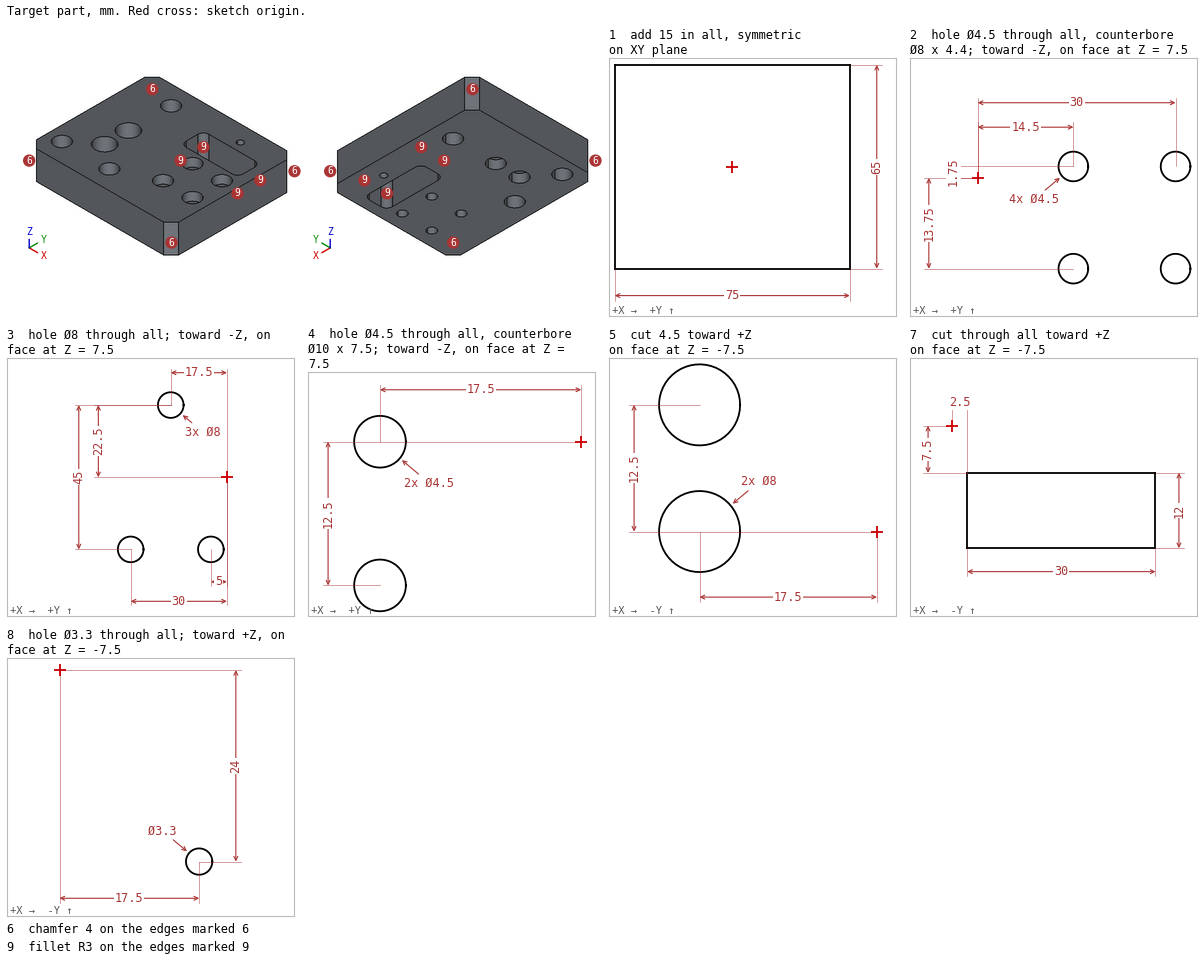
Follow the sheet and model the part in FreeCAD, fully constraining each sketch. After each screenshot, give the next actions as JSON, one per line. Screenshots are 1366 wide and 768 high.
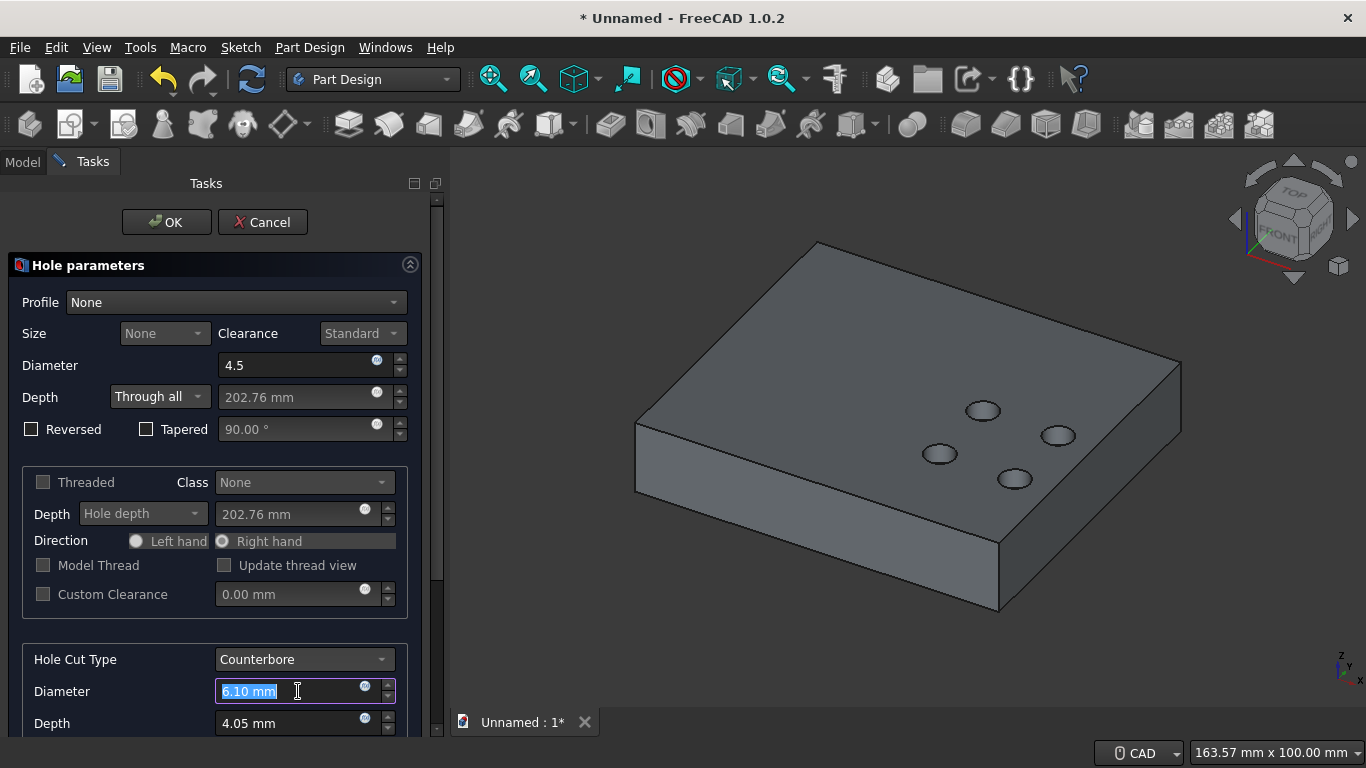
{"action": "type", "text": "8"}
{"action": "key", "text": "Tab"}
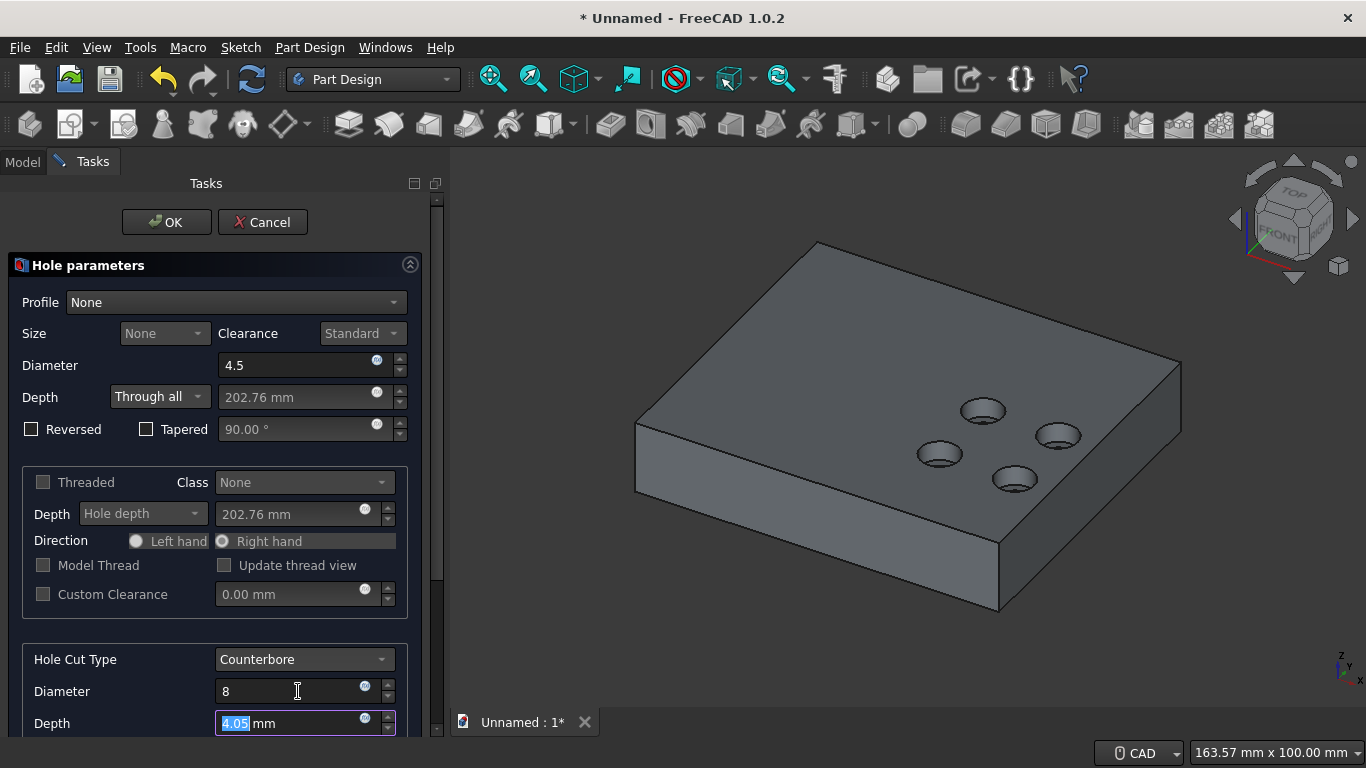
{"action": "type", "text": "4.4"}
{"action": "key", "text": "Tab"}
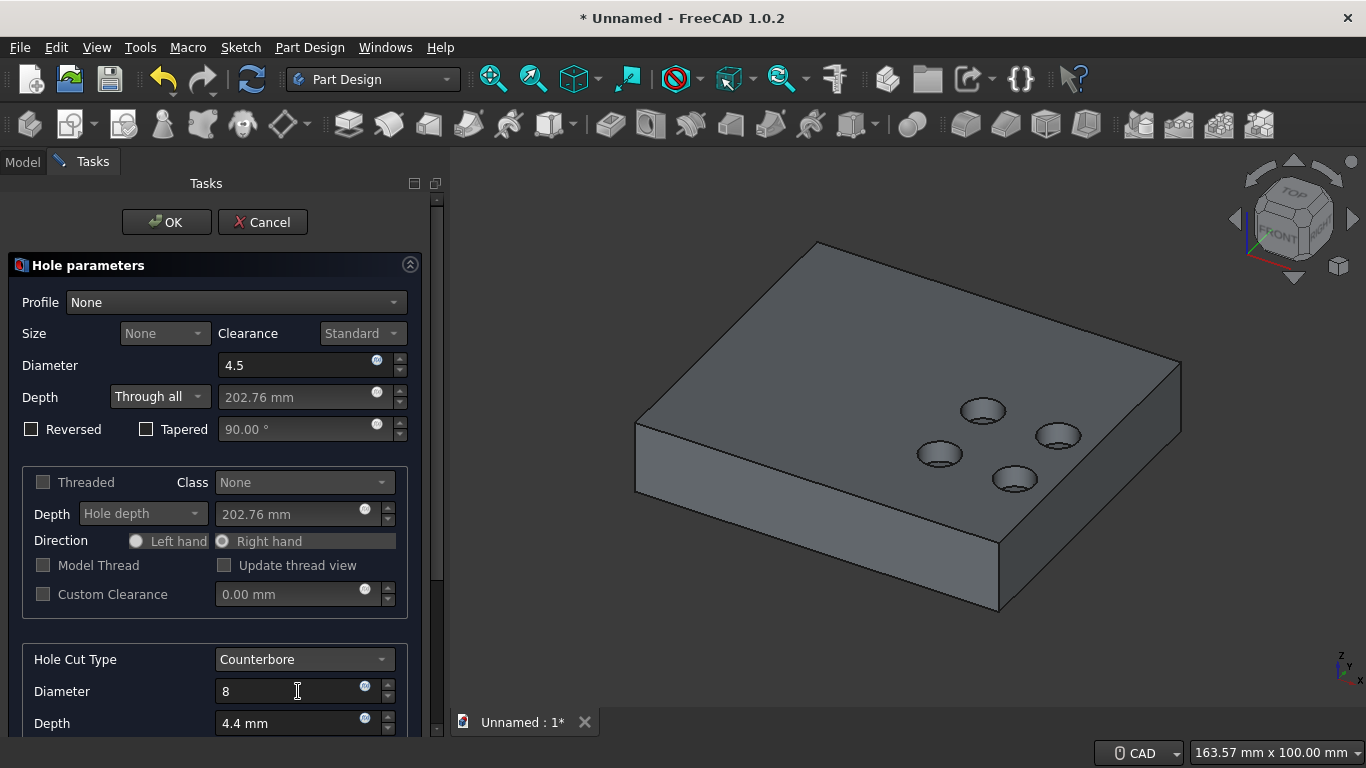
{"action": "left_click", "coordinate": [167, 222]}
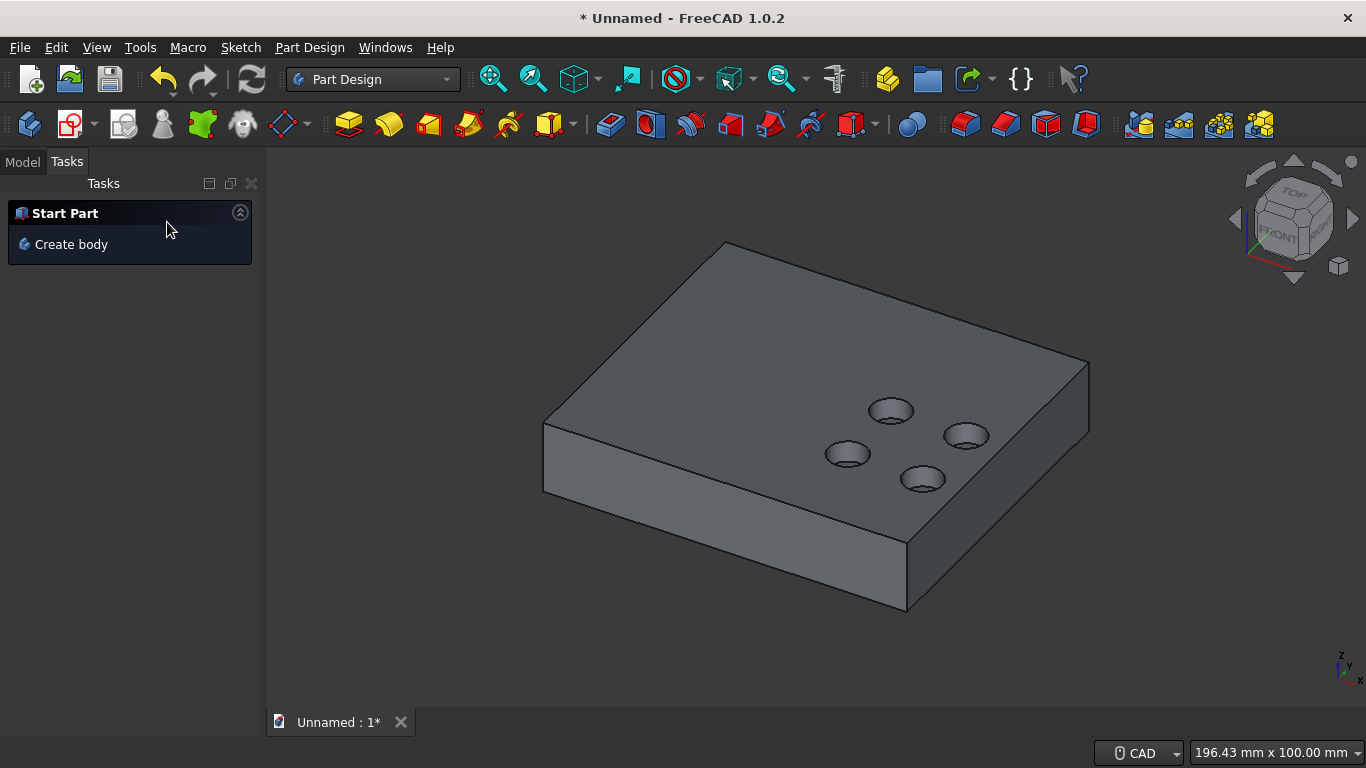
{"action": "left_click", "coordinate": [790, 349]}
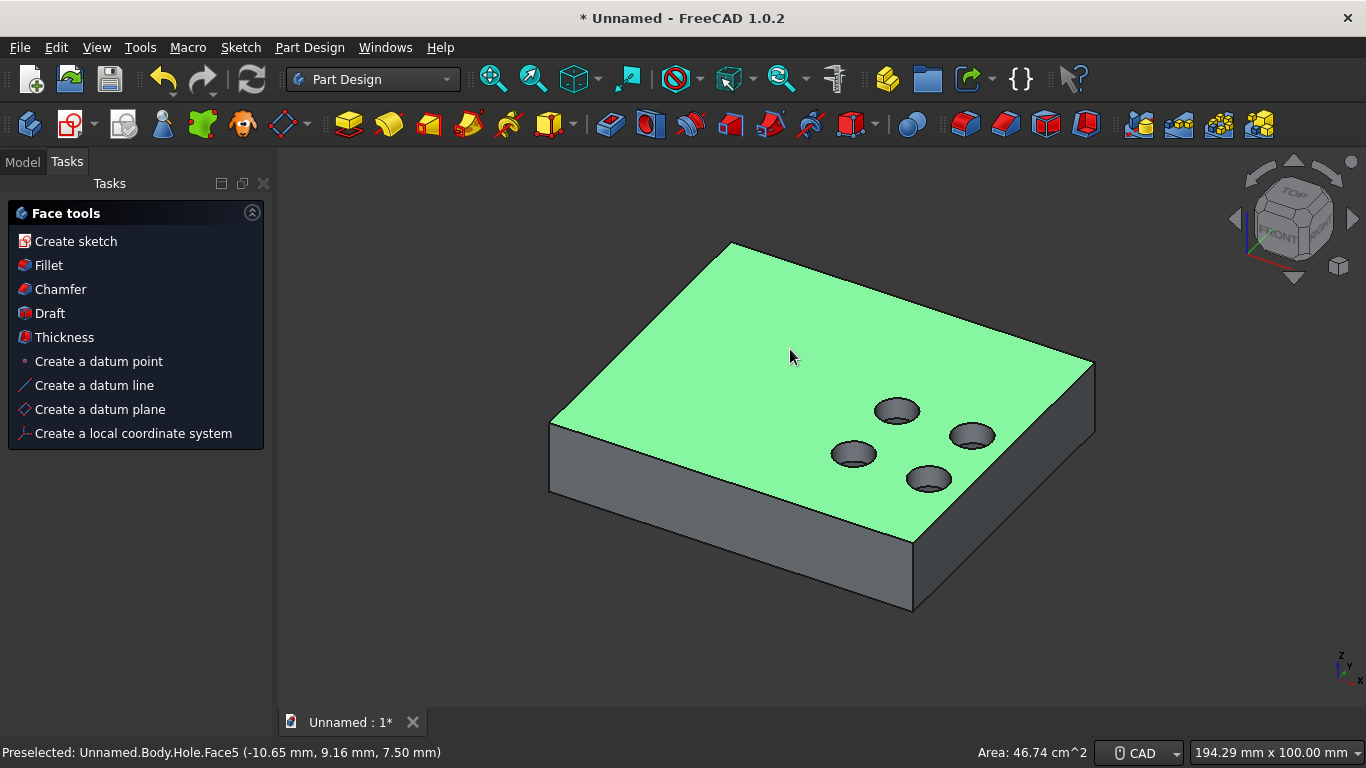
{"action": "left_click", "coordinate": [70, 124]}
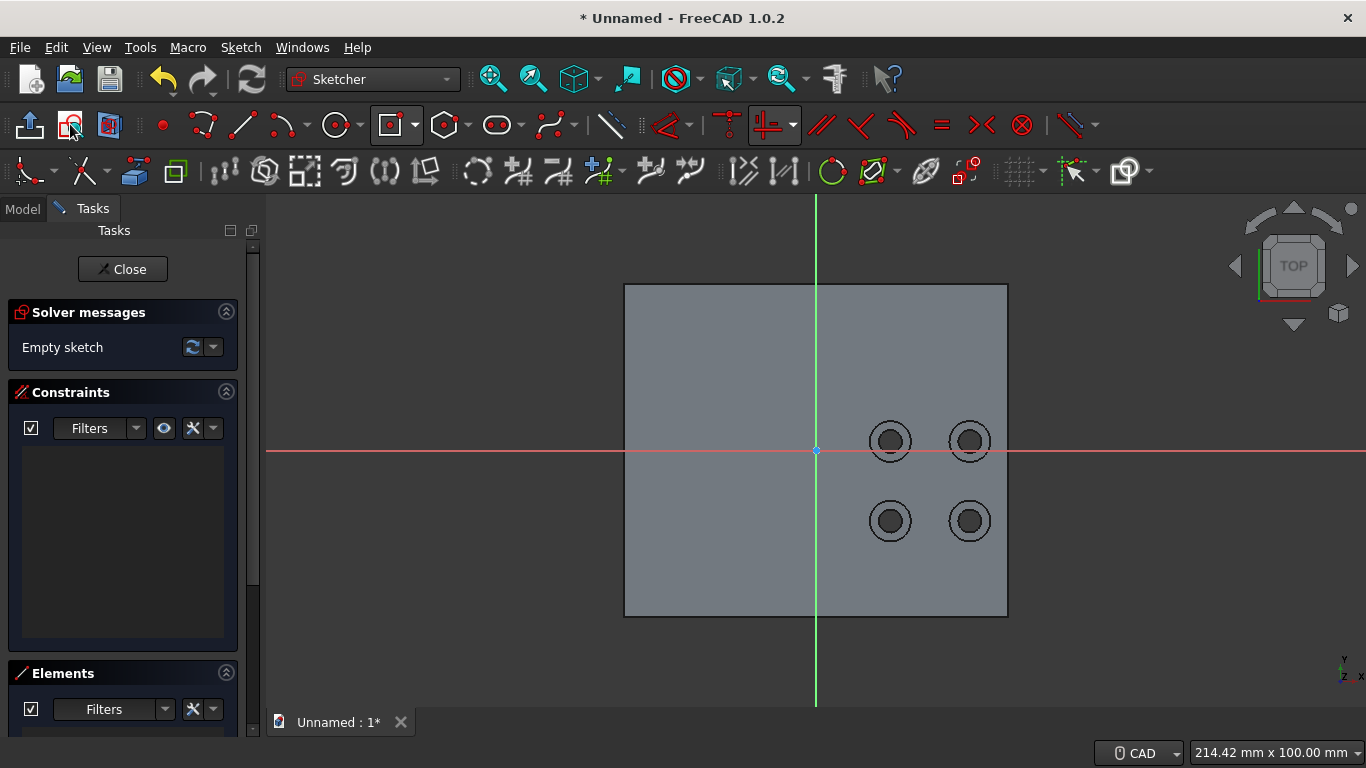
{"action": "key", "text": "g c"}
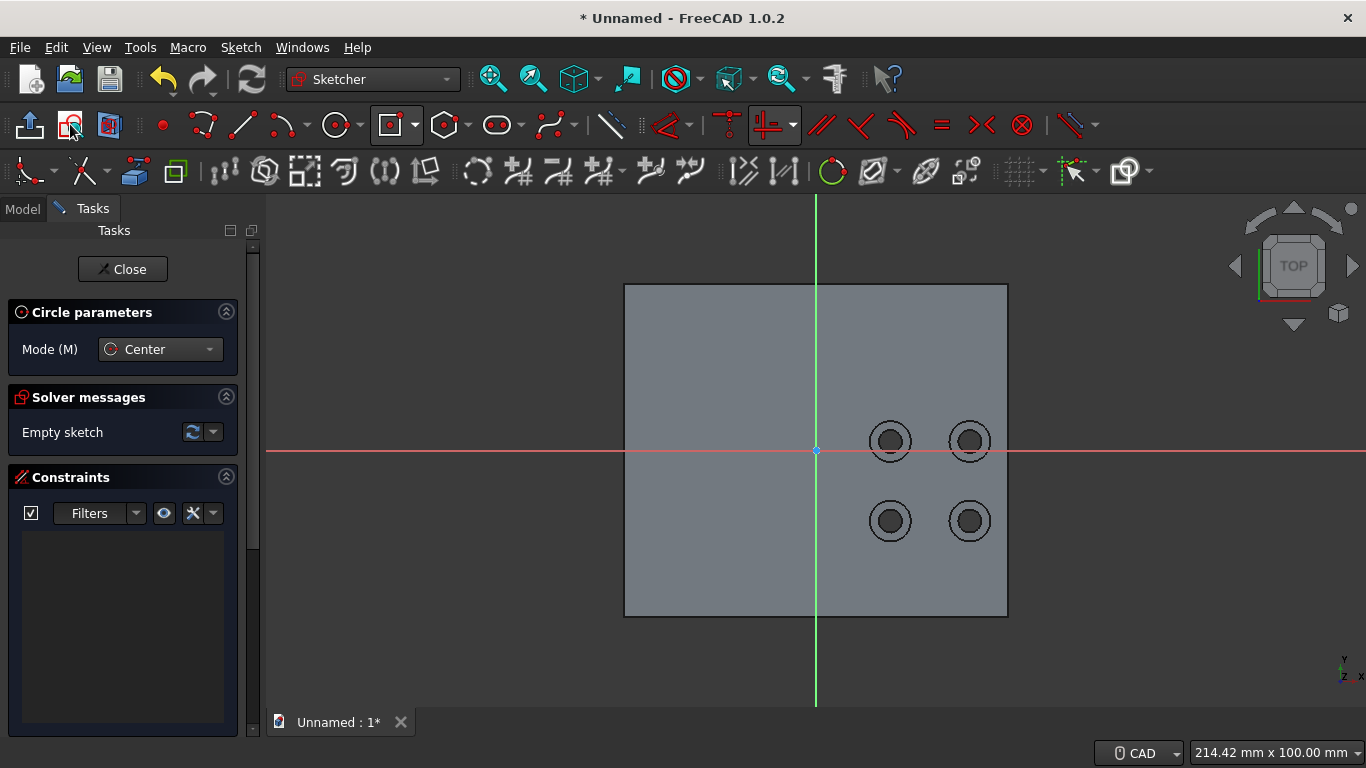
{"action": "left_click", "coordinate": [726, 335]}
{"action": "mouse_move", "coordinate": [741, 321]}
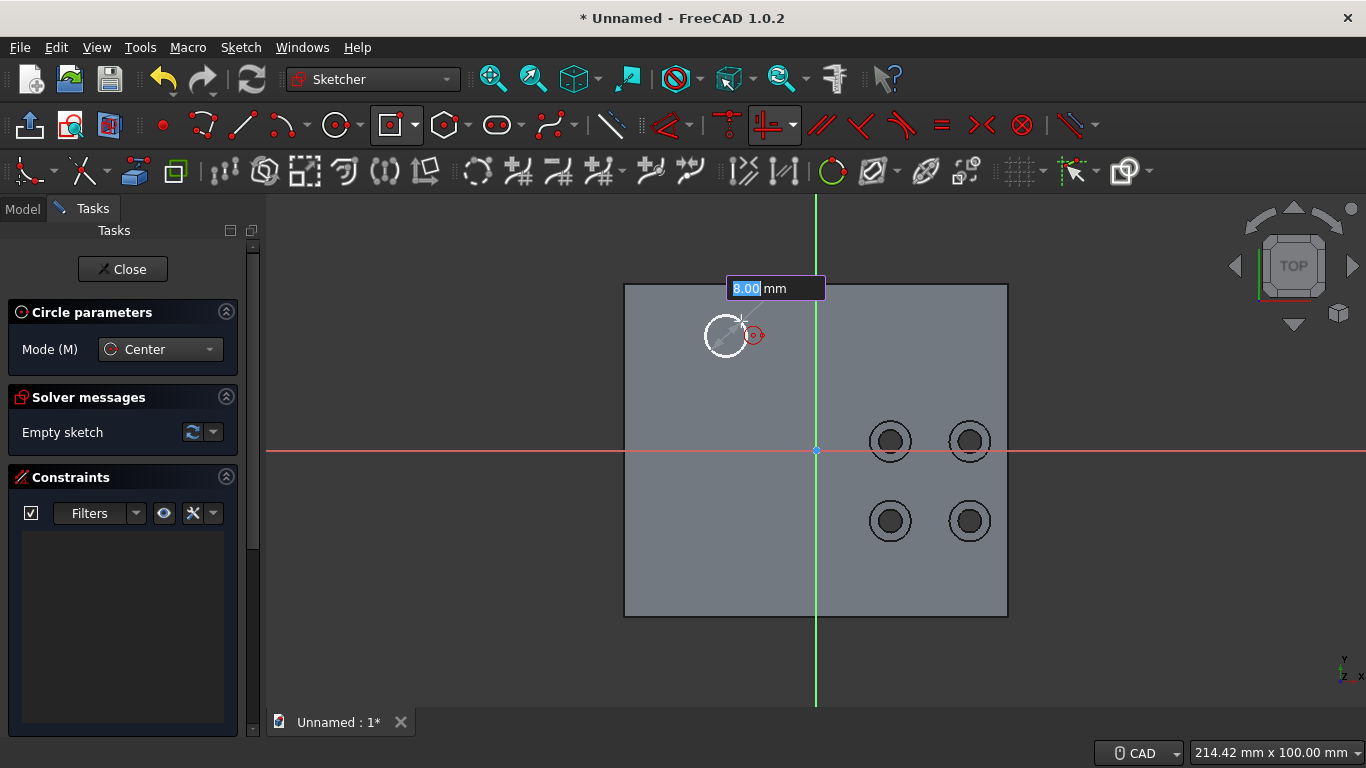
{"action": "type", "text": "8"}
{"action": "key", "text": "Return"}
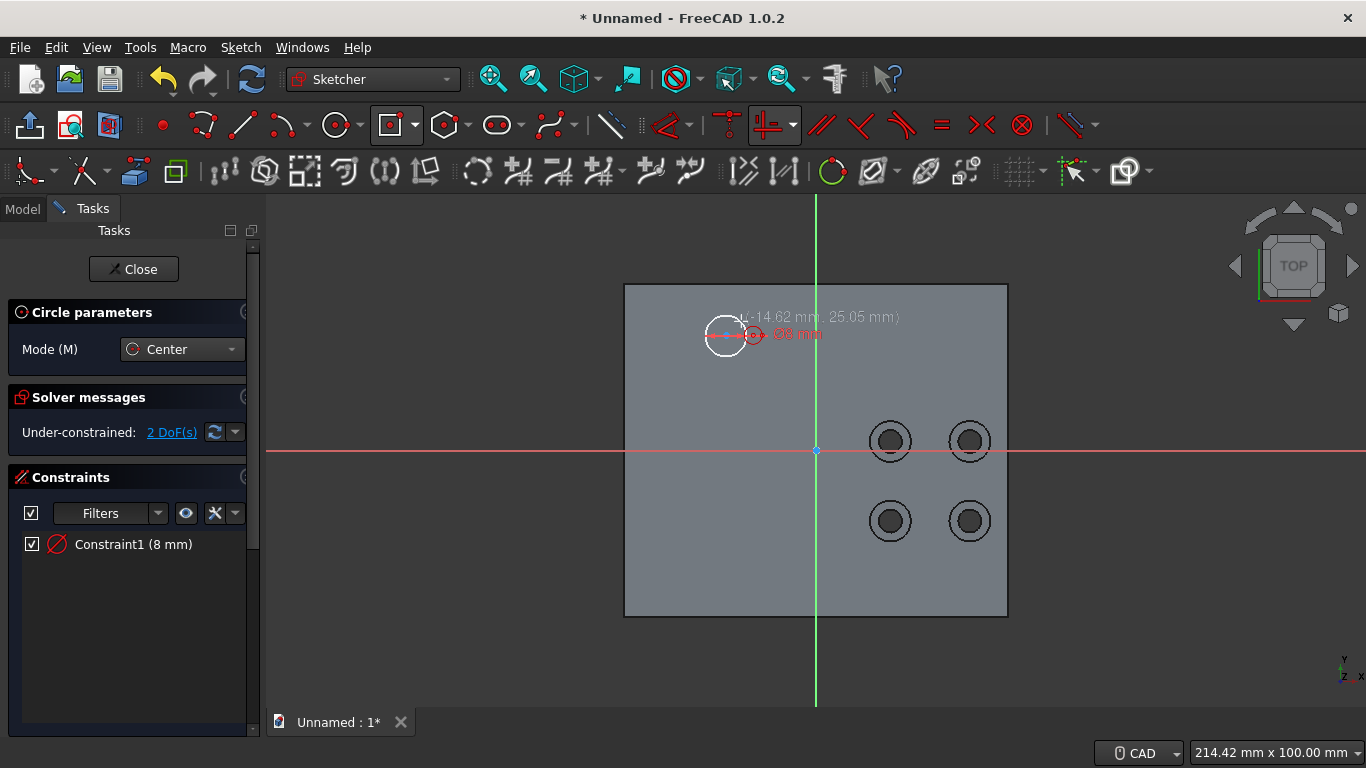
{"action": "left_click", "coordinate": [662, 566]}
{"action": "mouse_move", "coordinate": [677, 551]}